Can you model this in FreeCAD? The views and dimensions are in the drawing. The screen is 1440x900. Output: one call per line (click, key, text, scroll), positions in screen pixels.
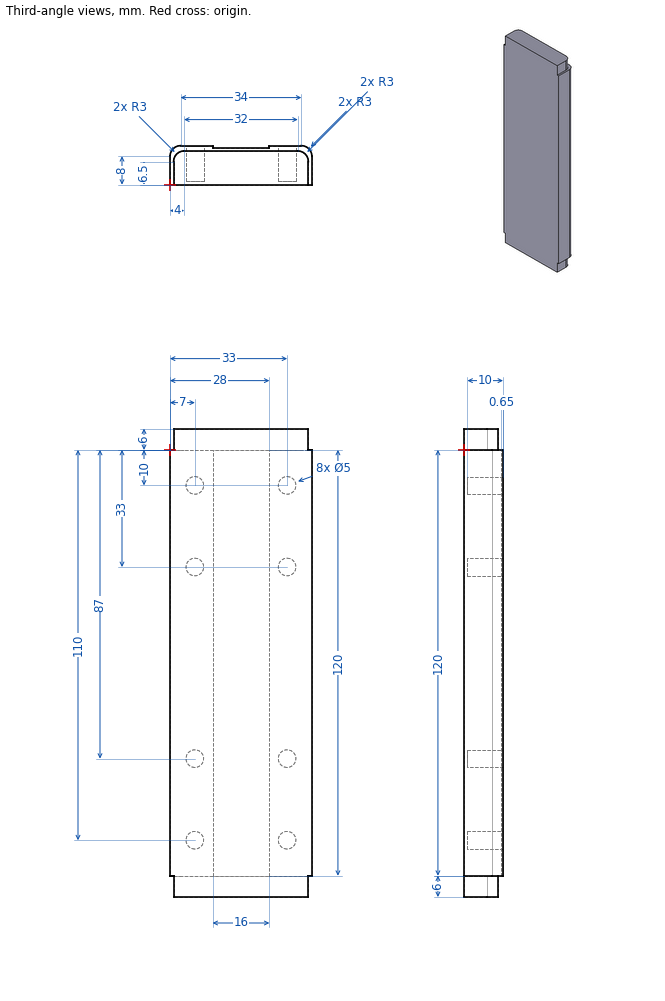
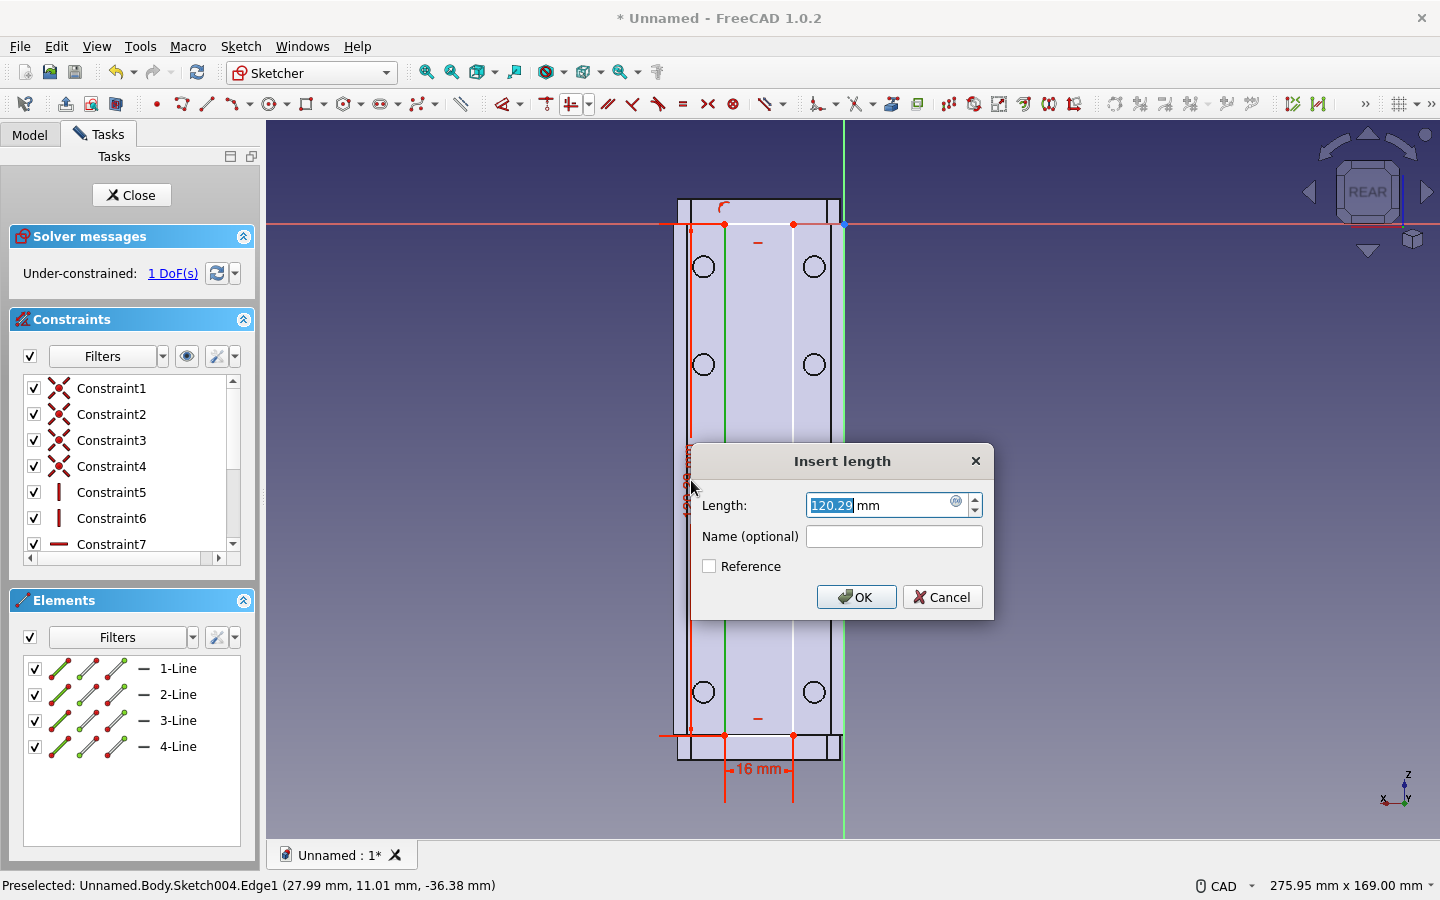
text(120)
key(Return)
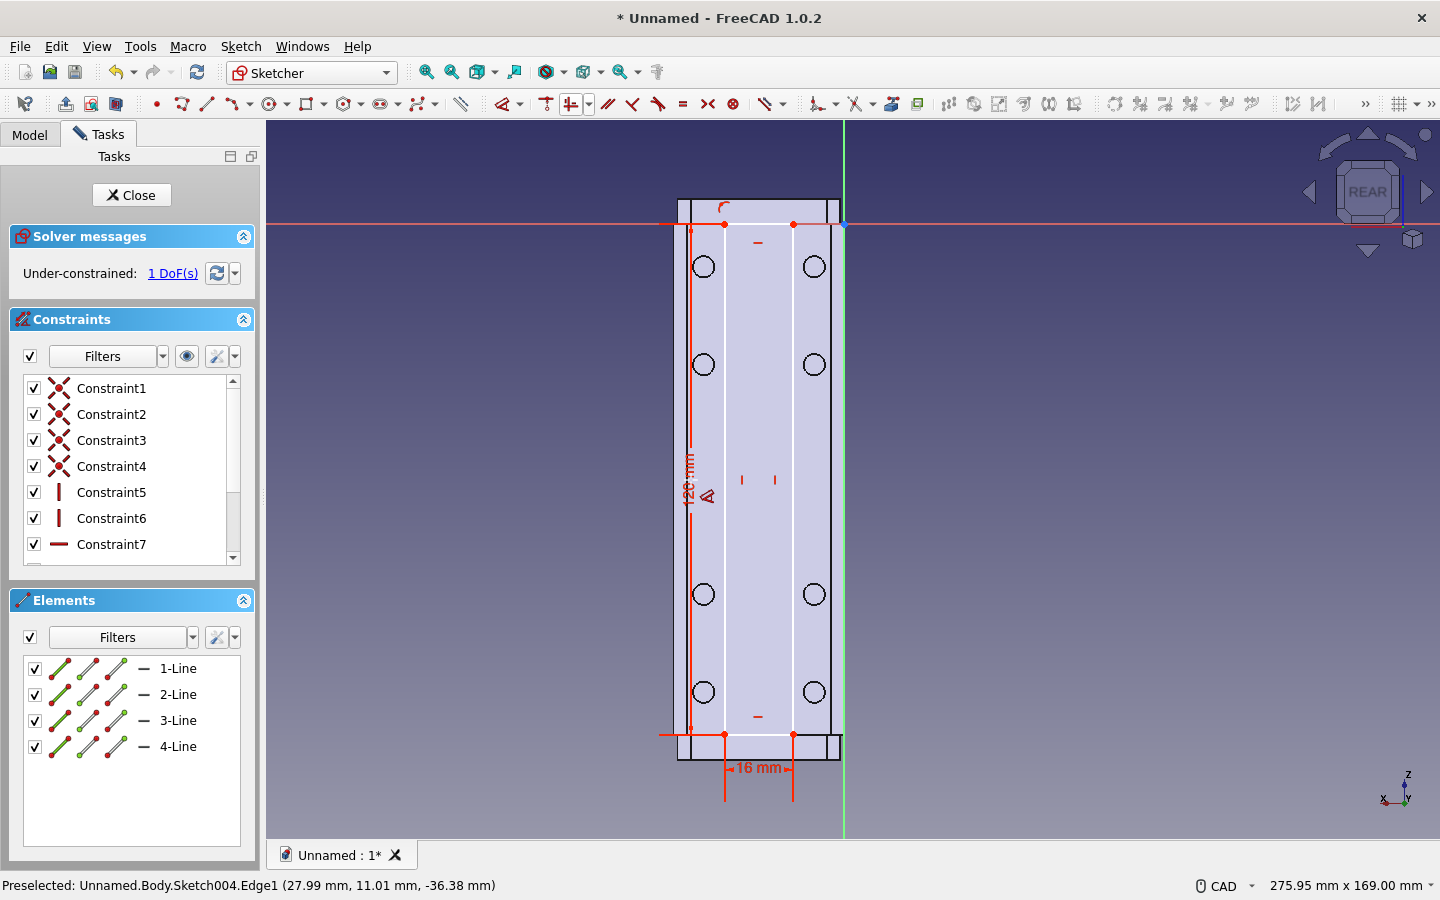
click(725, 224)
click(784, 190)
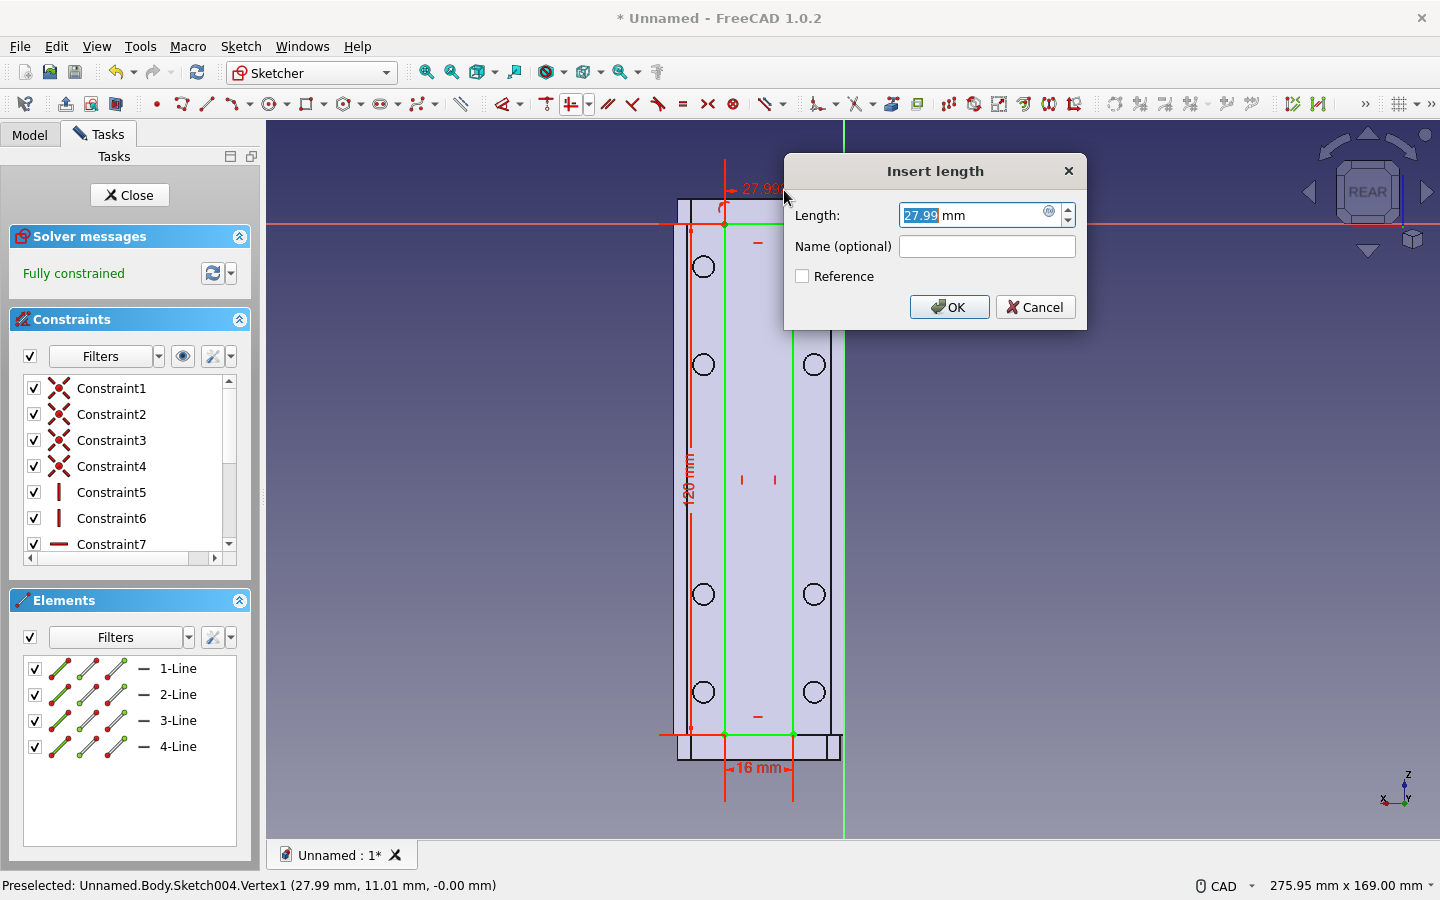
text(28)
key(Return)
key(Escape)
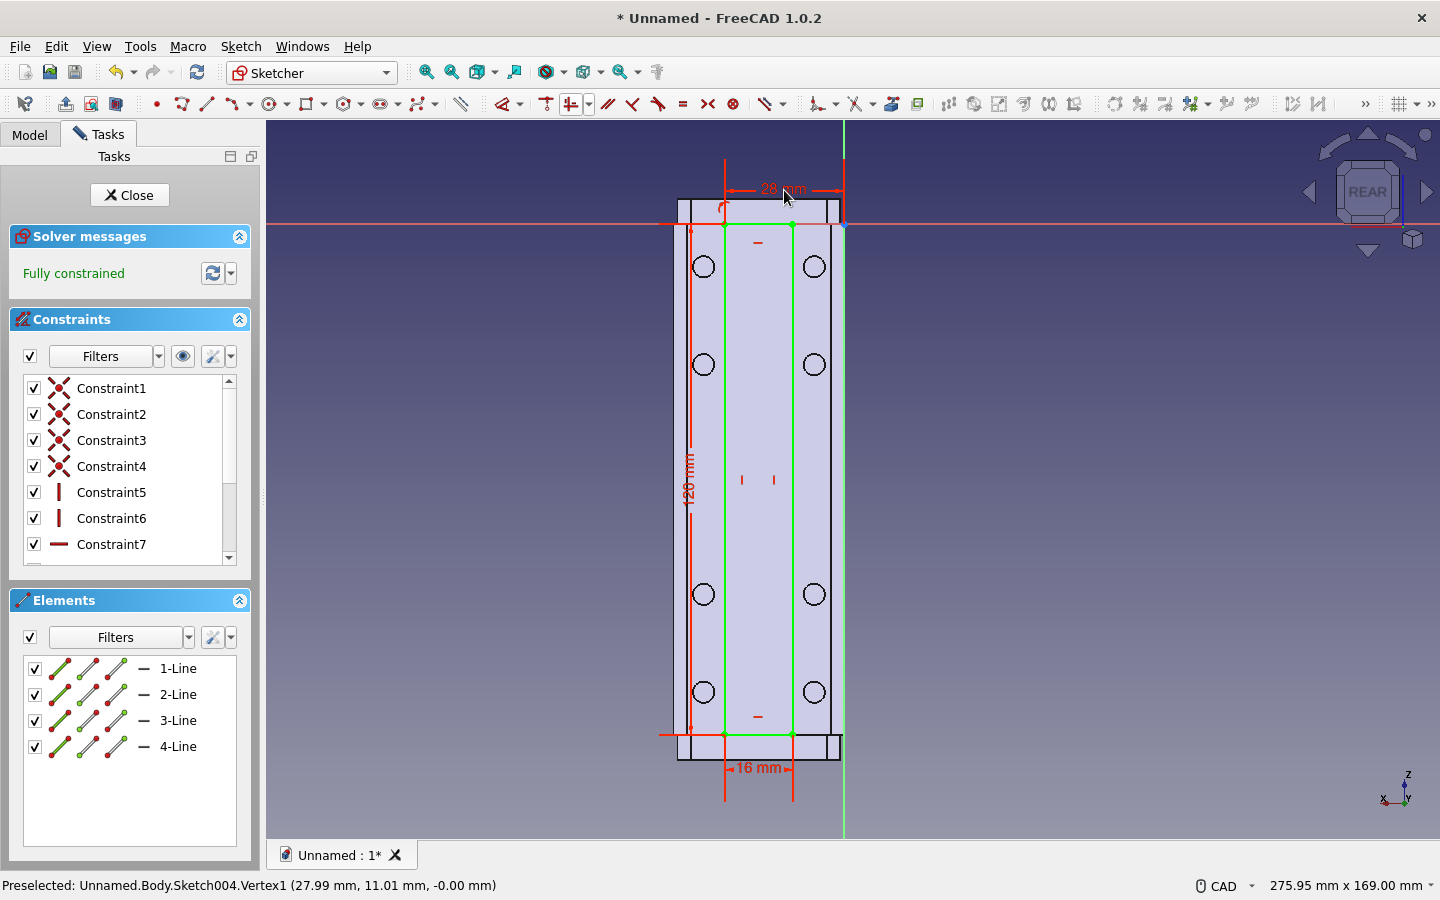
click(130, 195)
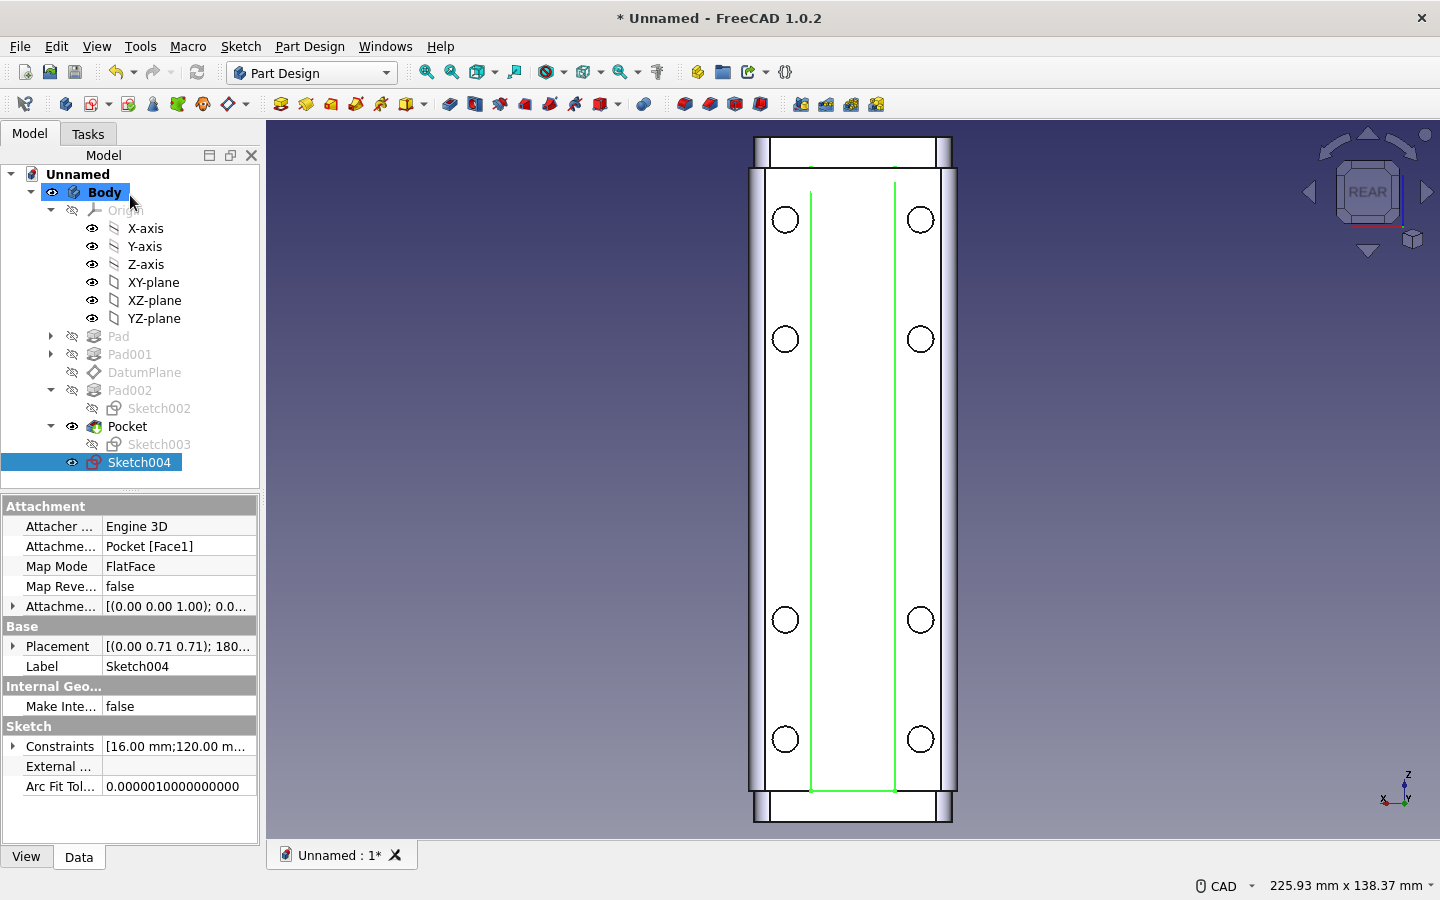
click(450, 104)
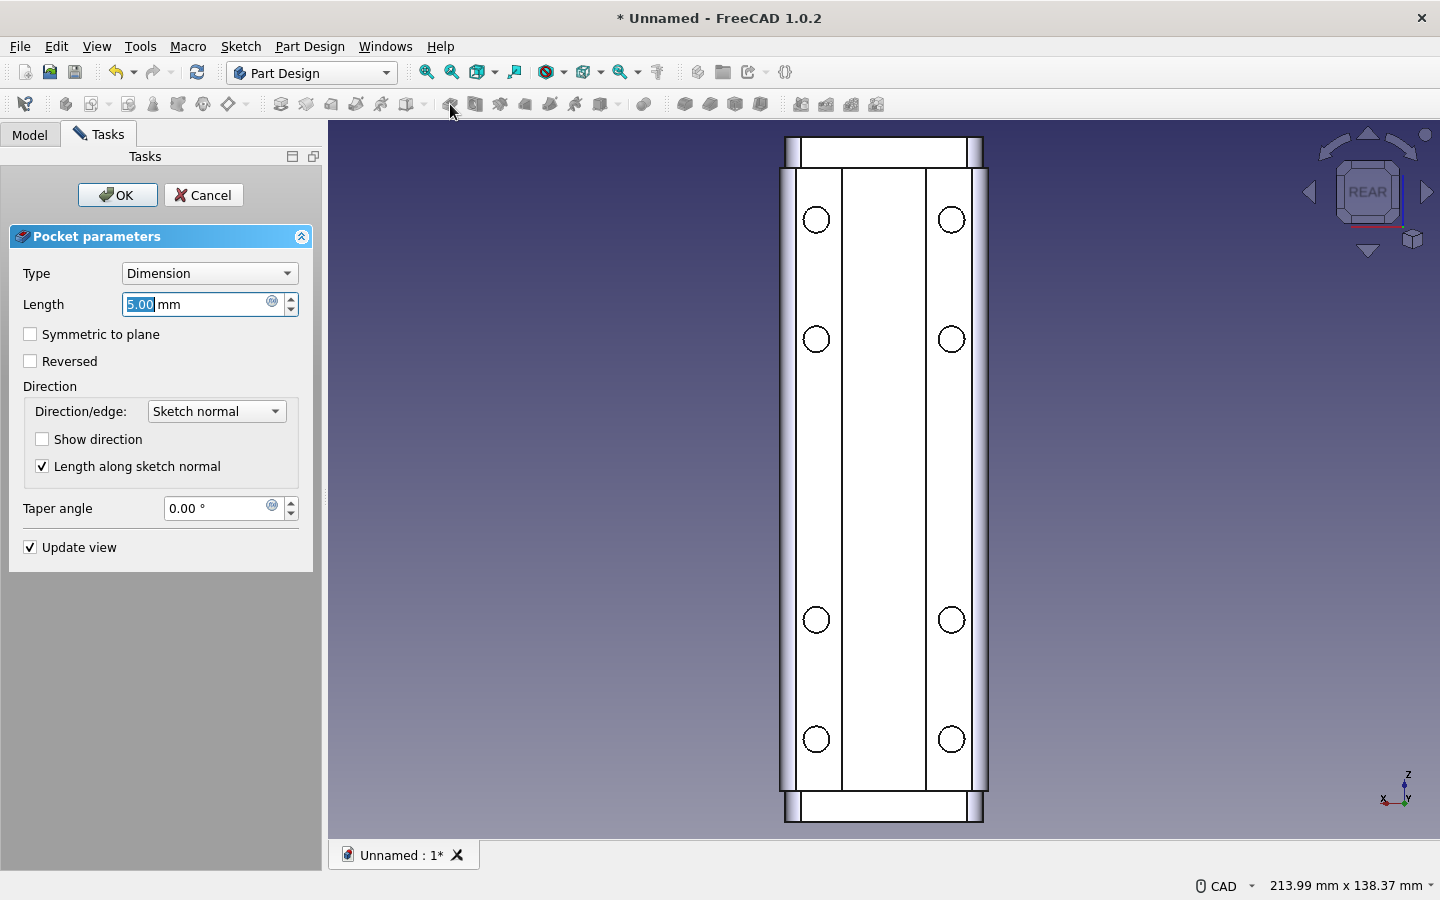
text(0.65)
key(Tab)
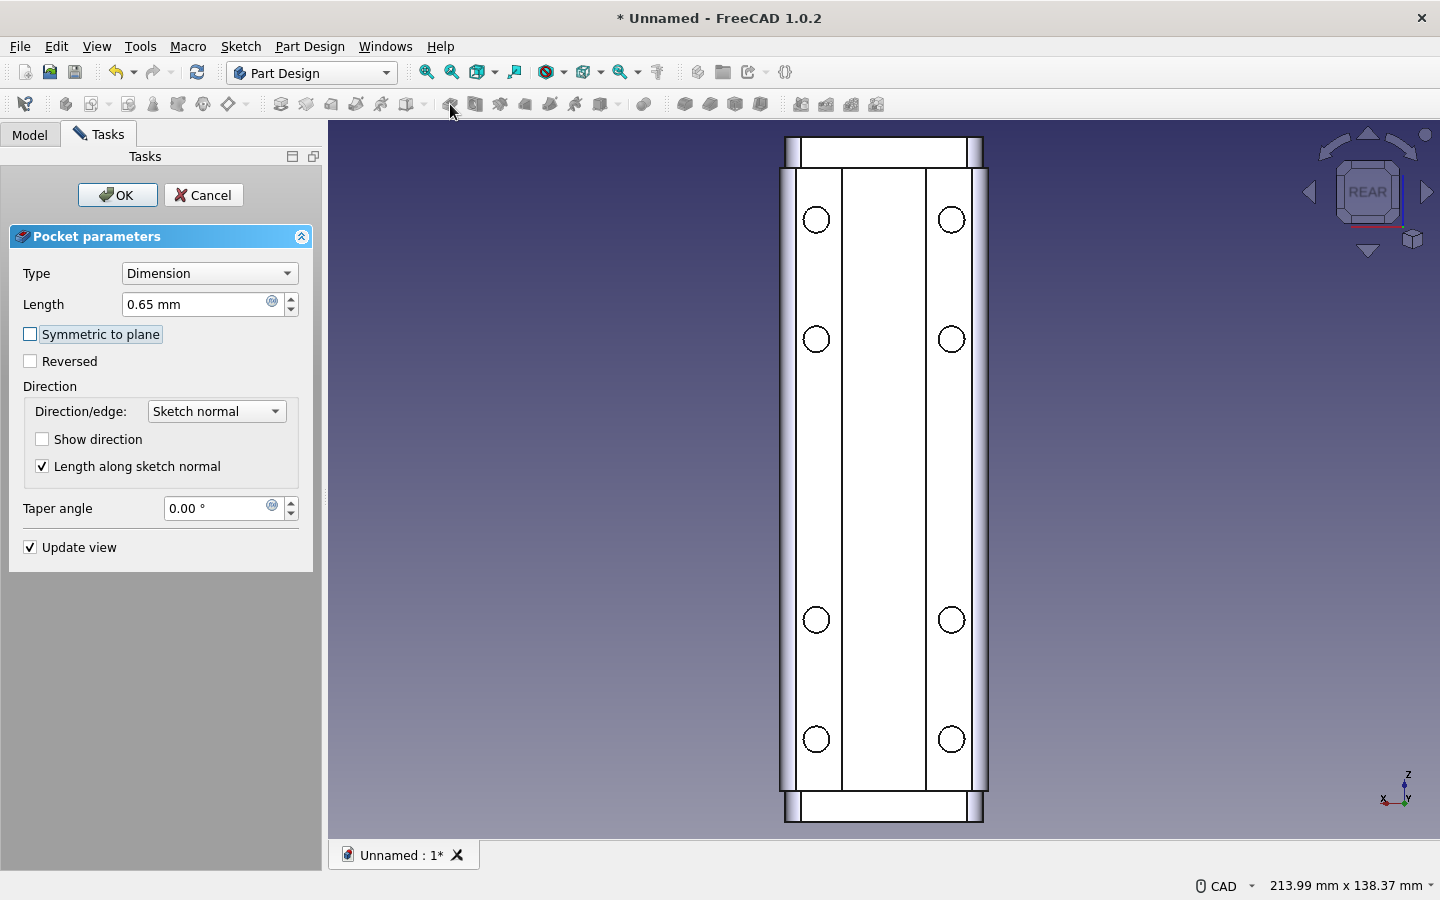
click(118, 195)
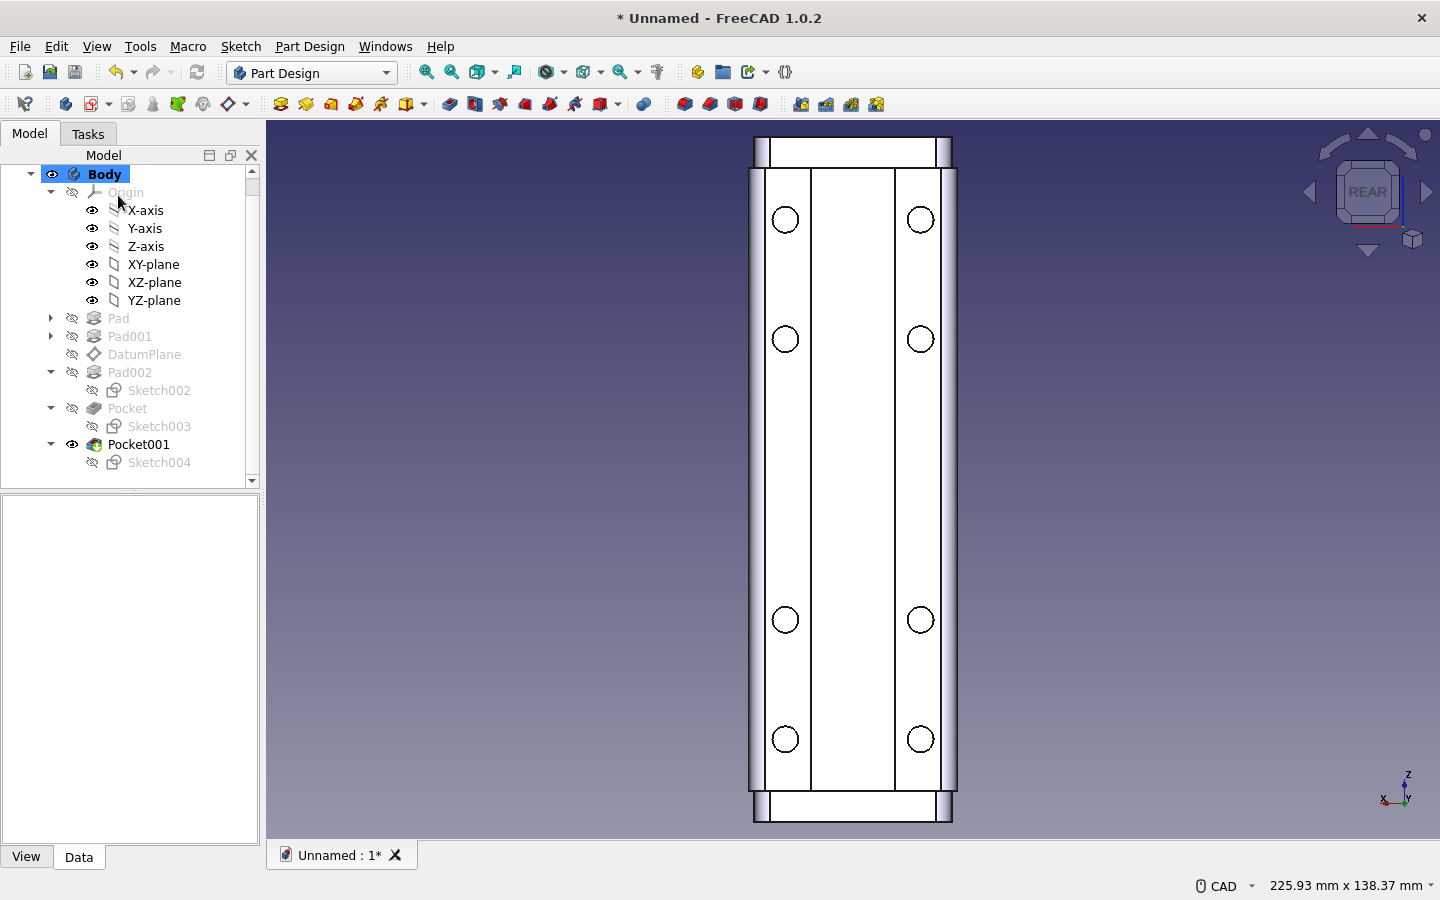
key(0)